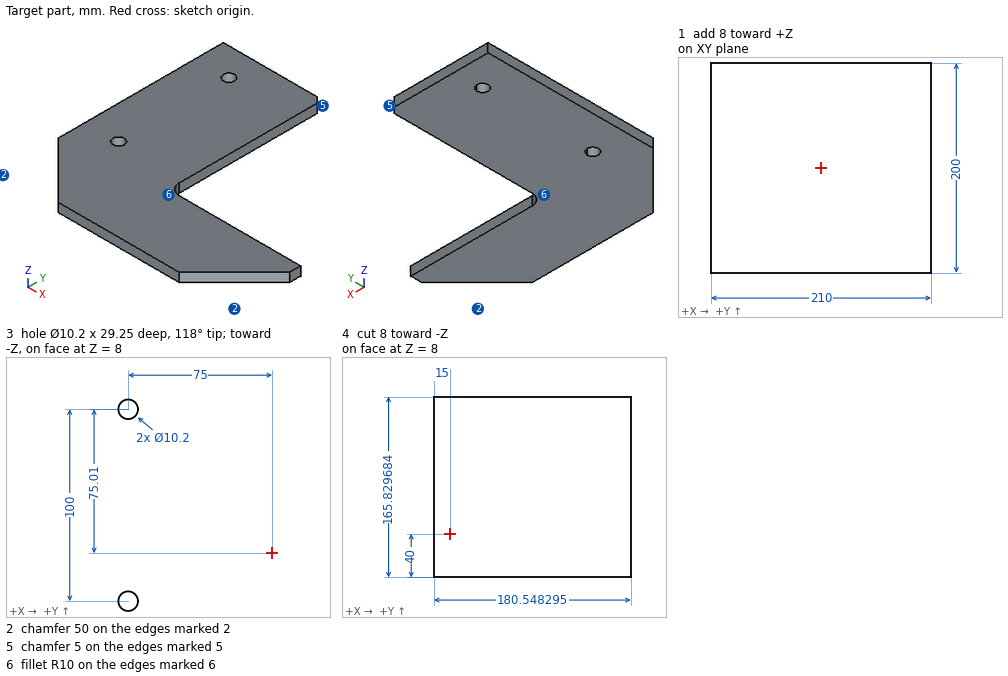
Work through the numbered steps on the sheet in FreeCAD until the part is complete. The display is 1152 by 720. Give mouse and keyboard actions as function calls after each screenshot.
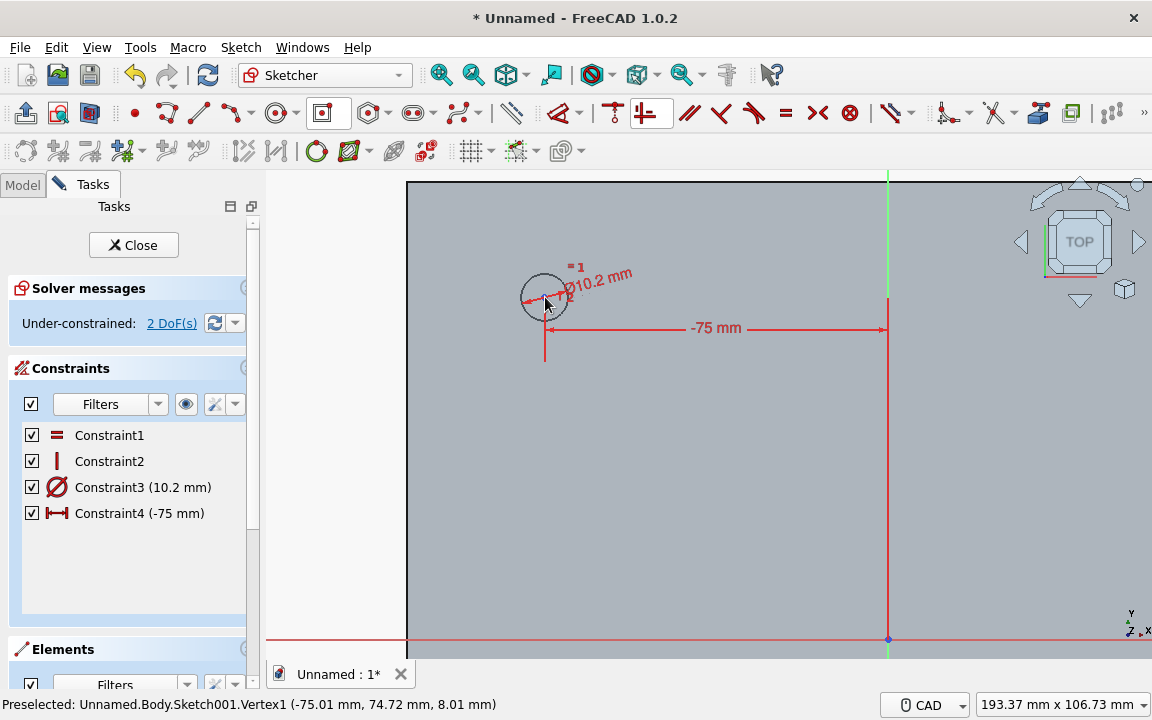
click(545, 297)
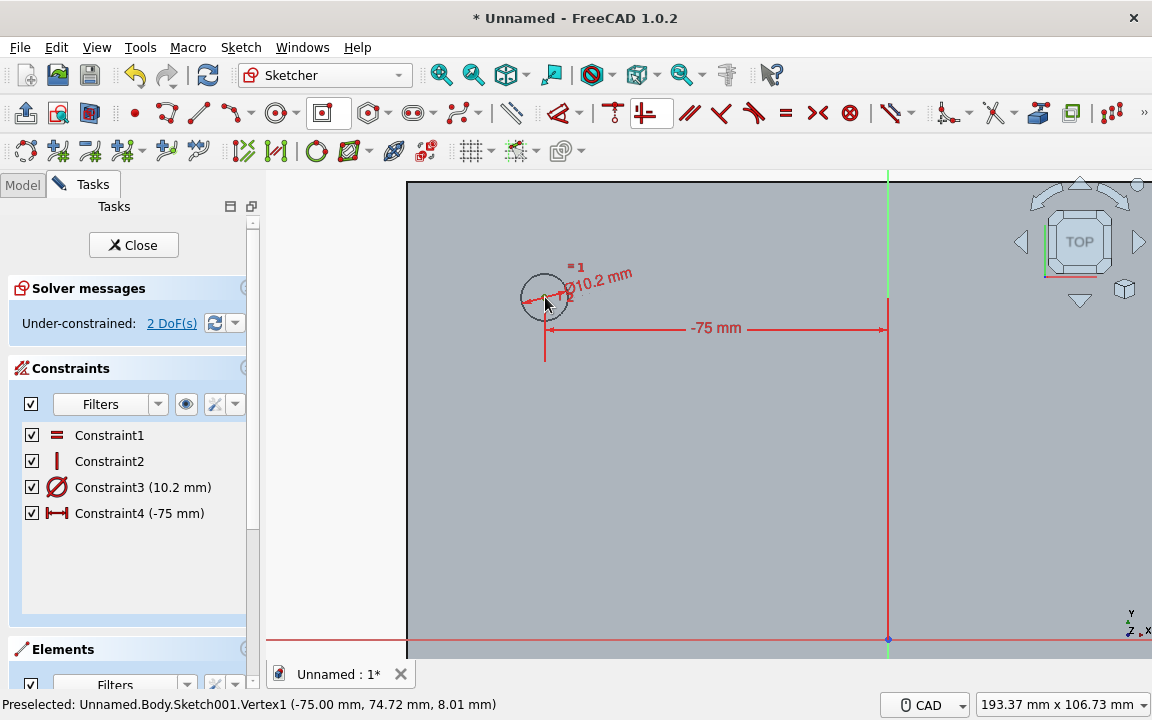
scroll(562, 280, down, 3)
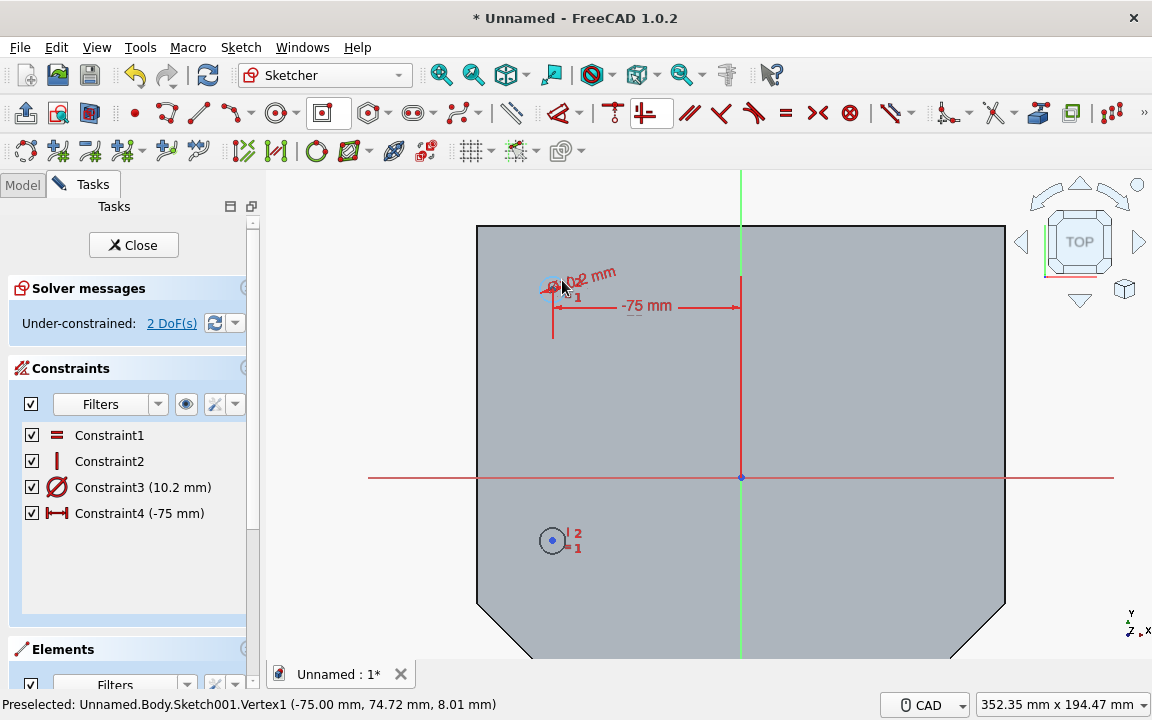
click(553, 541)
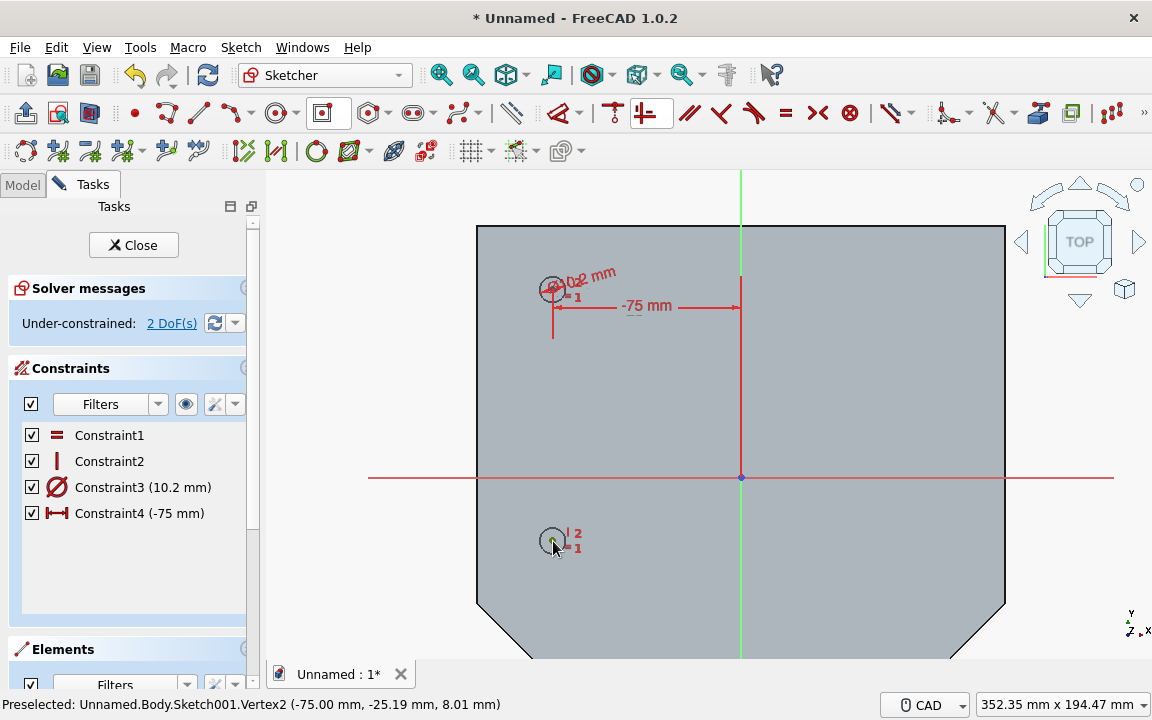
key(i)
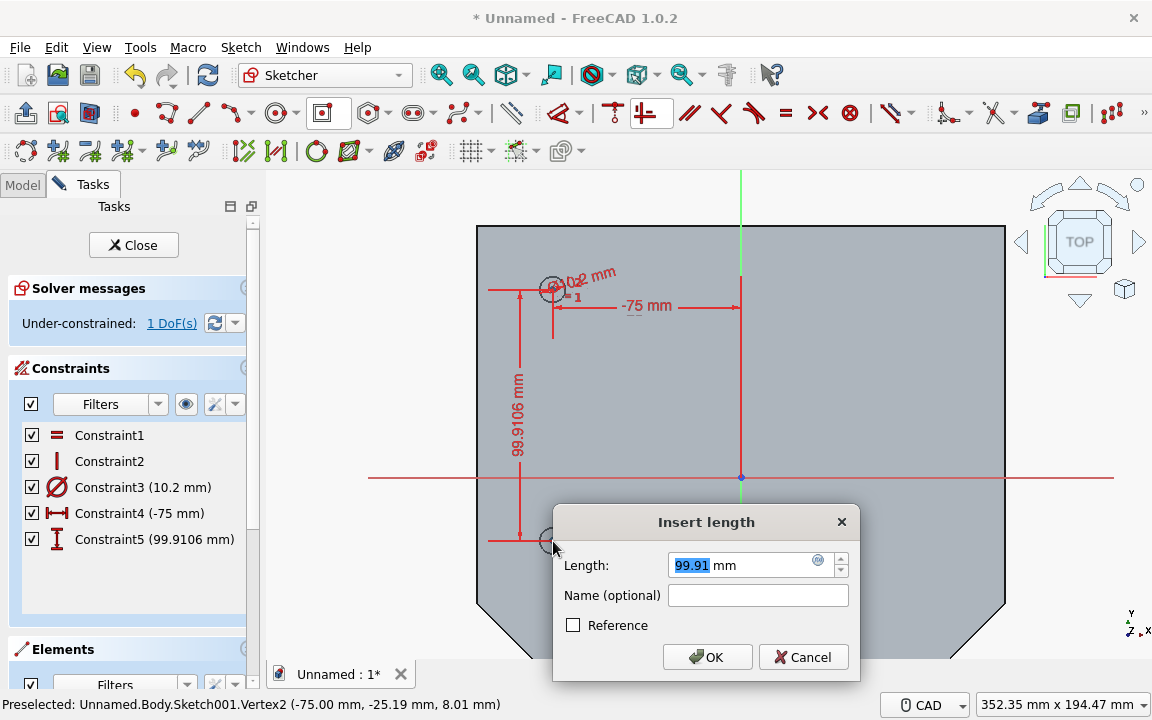
text(100)
key(Return)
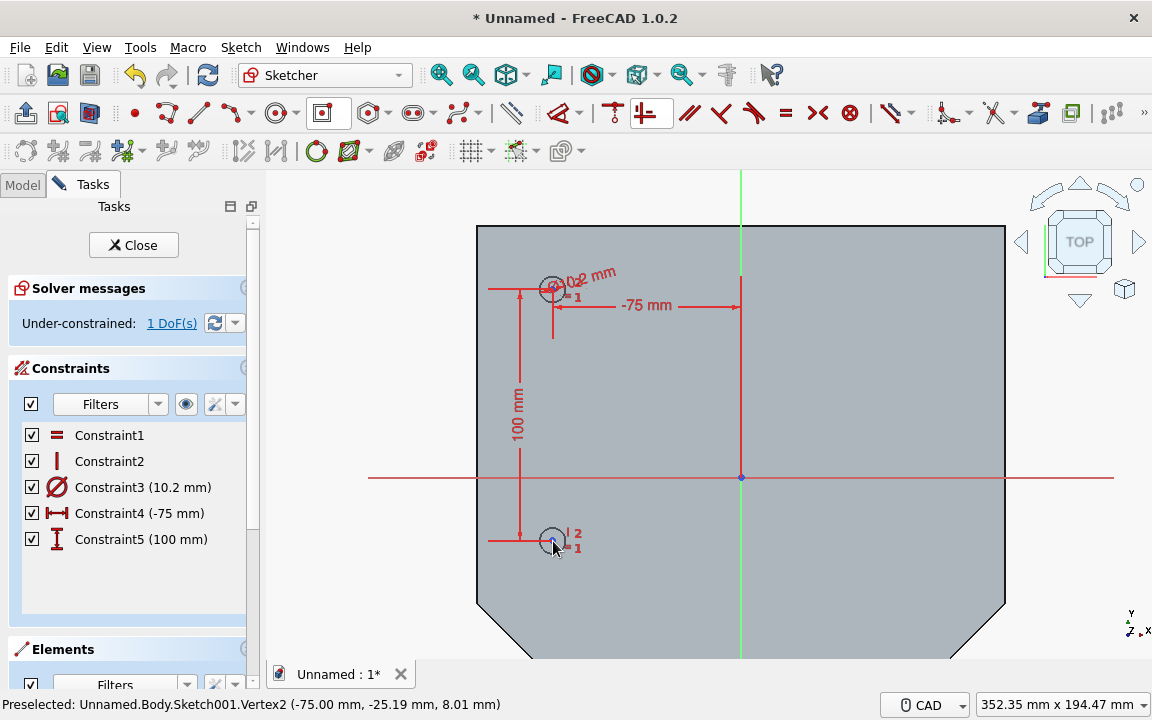
click(553, 289)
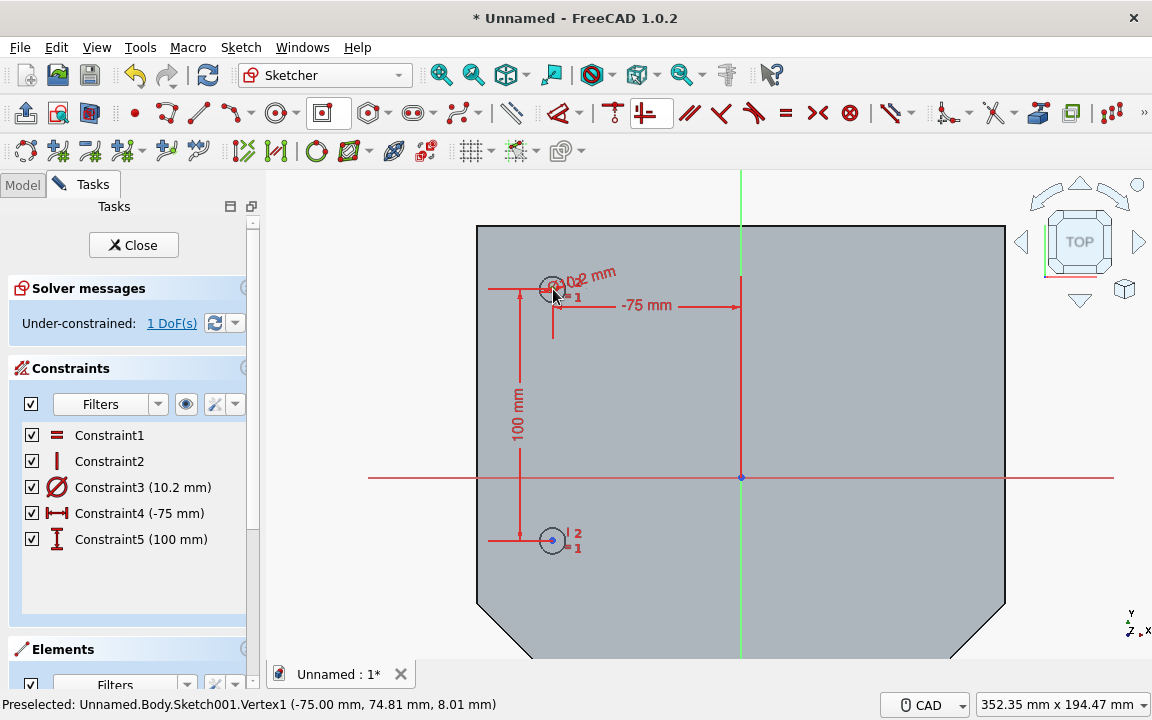
key(i)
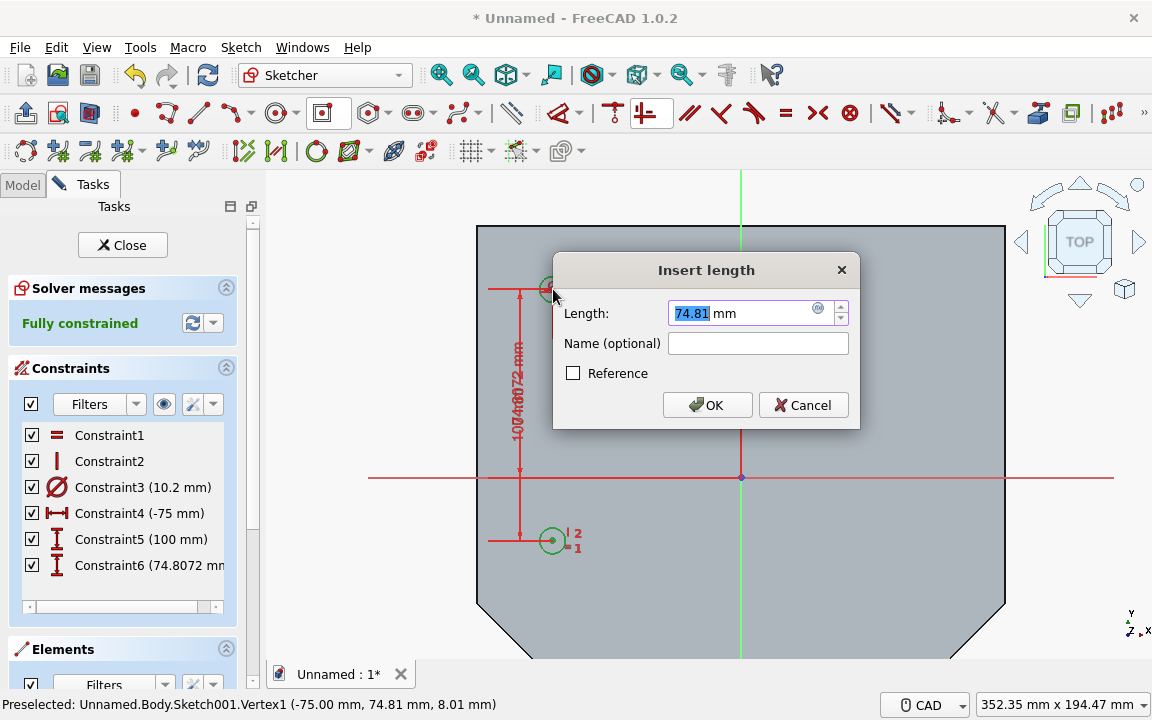
text(75.01)
key(Return)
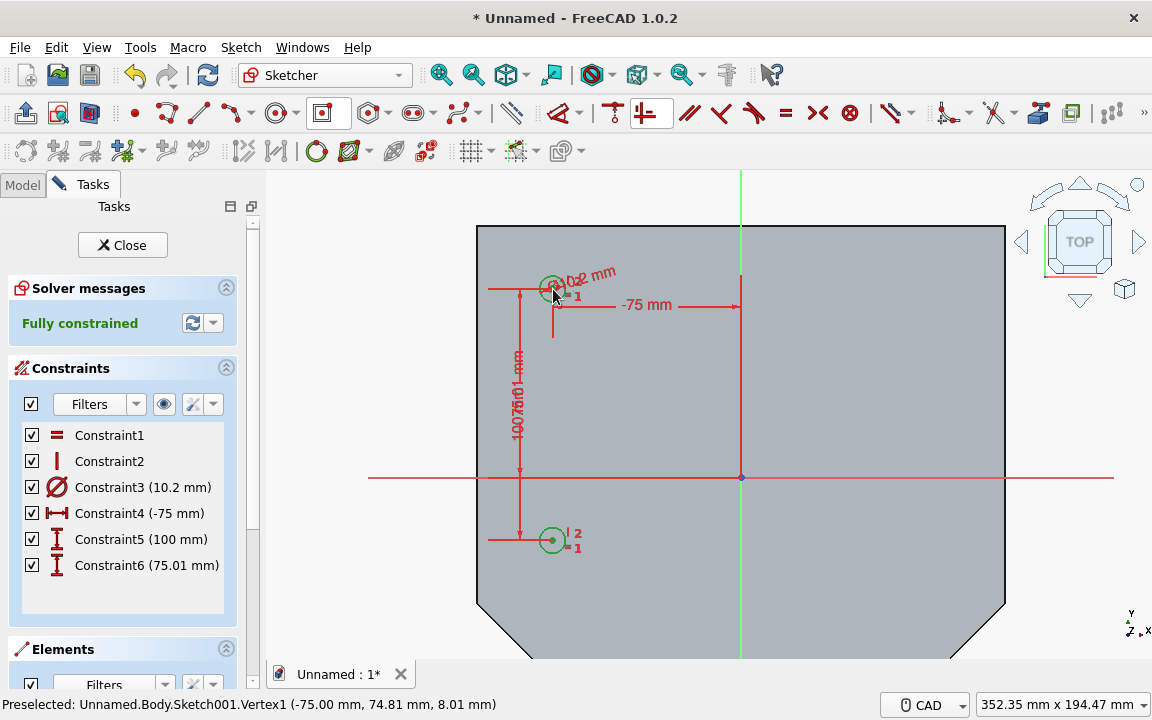
click(123, 245)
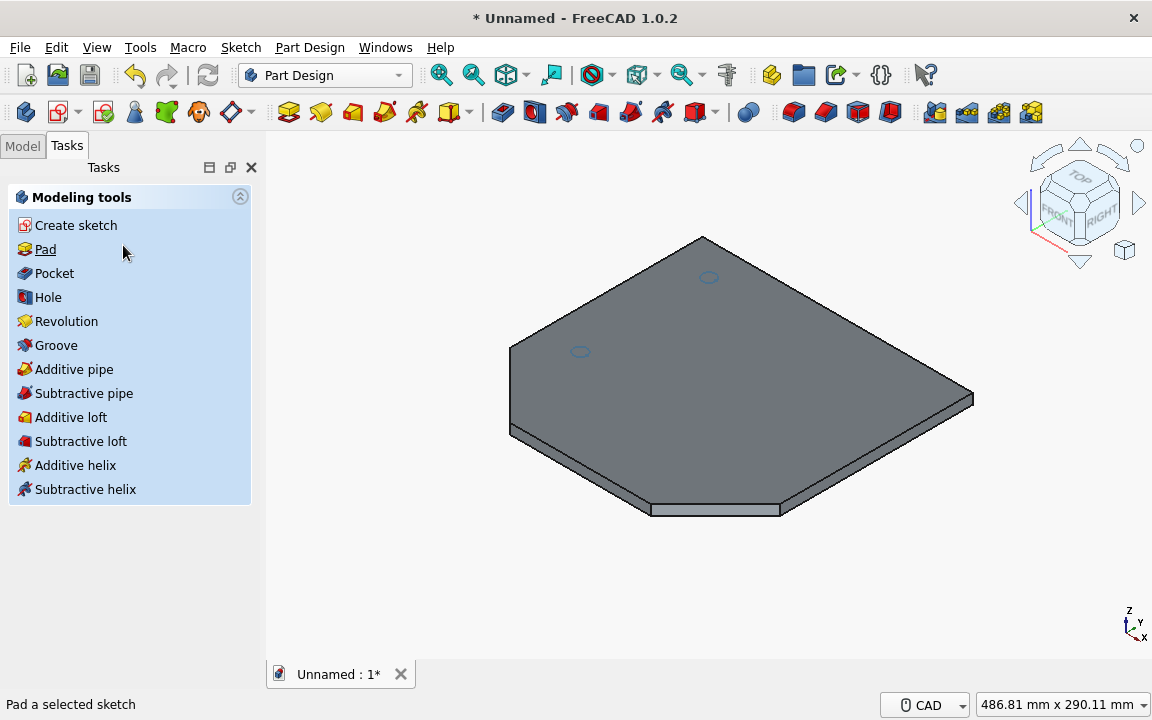
click(536, 112)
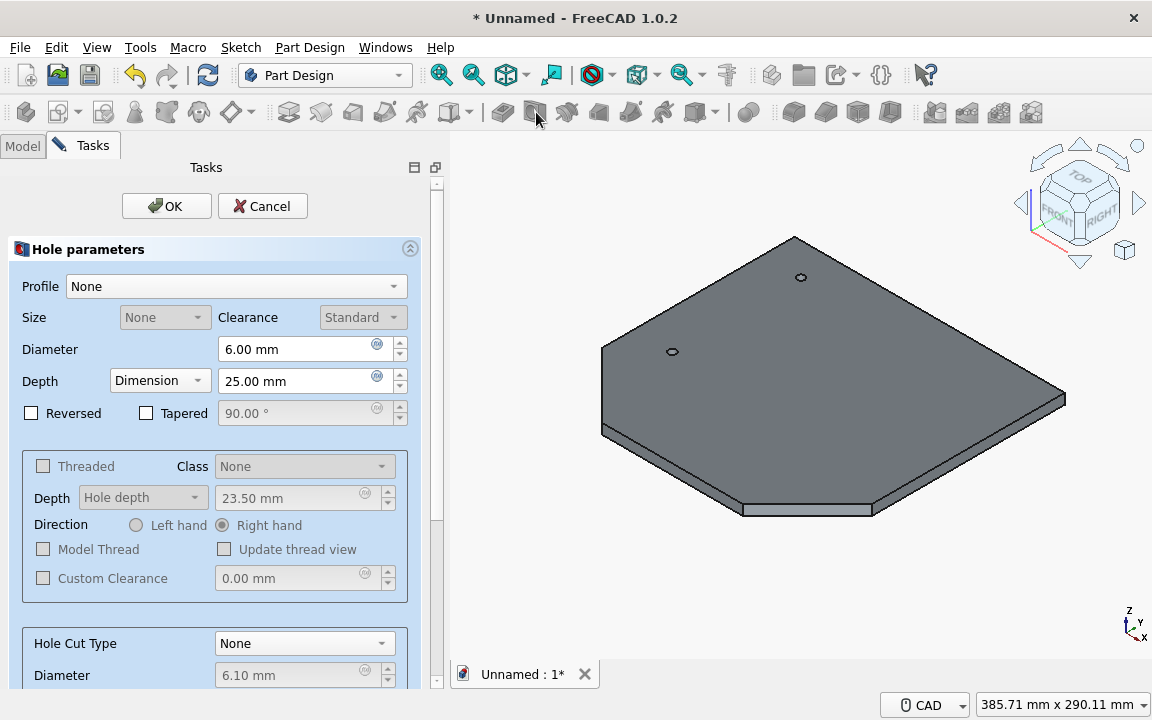
triple_click(305, 349)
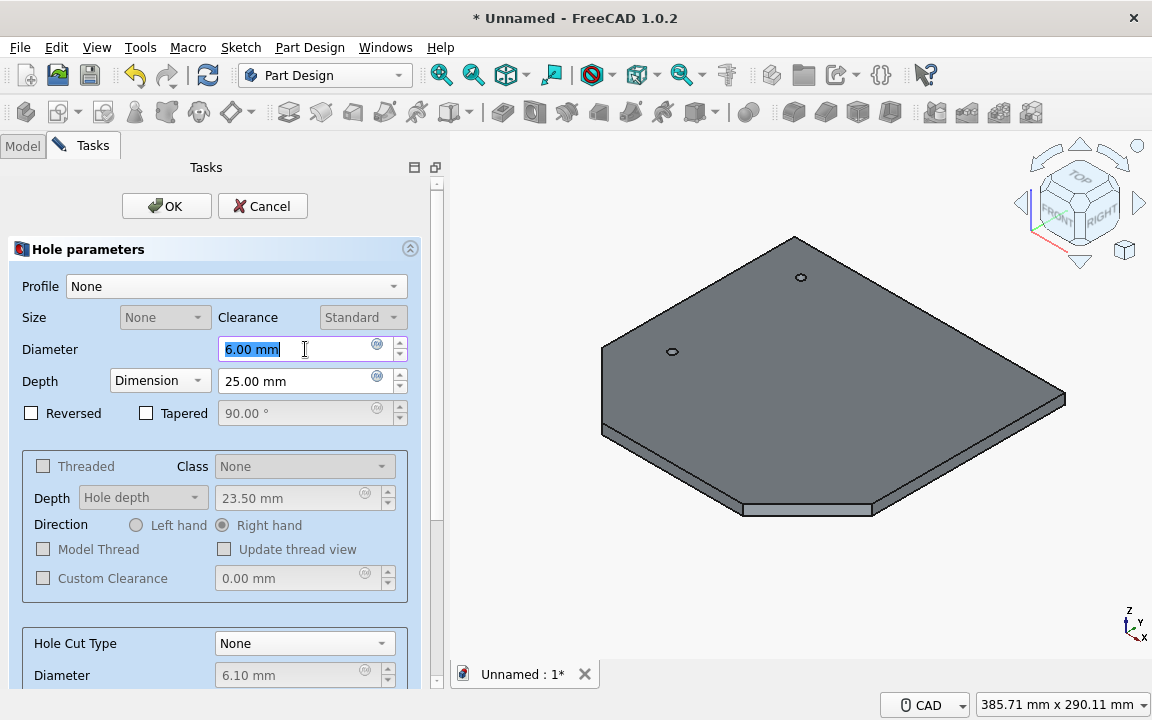
text(10.2)
key(Tab)